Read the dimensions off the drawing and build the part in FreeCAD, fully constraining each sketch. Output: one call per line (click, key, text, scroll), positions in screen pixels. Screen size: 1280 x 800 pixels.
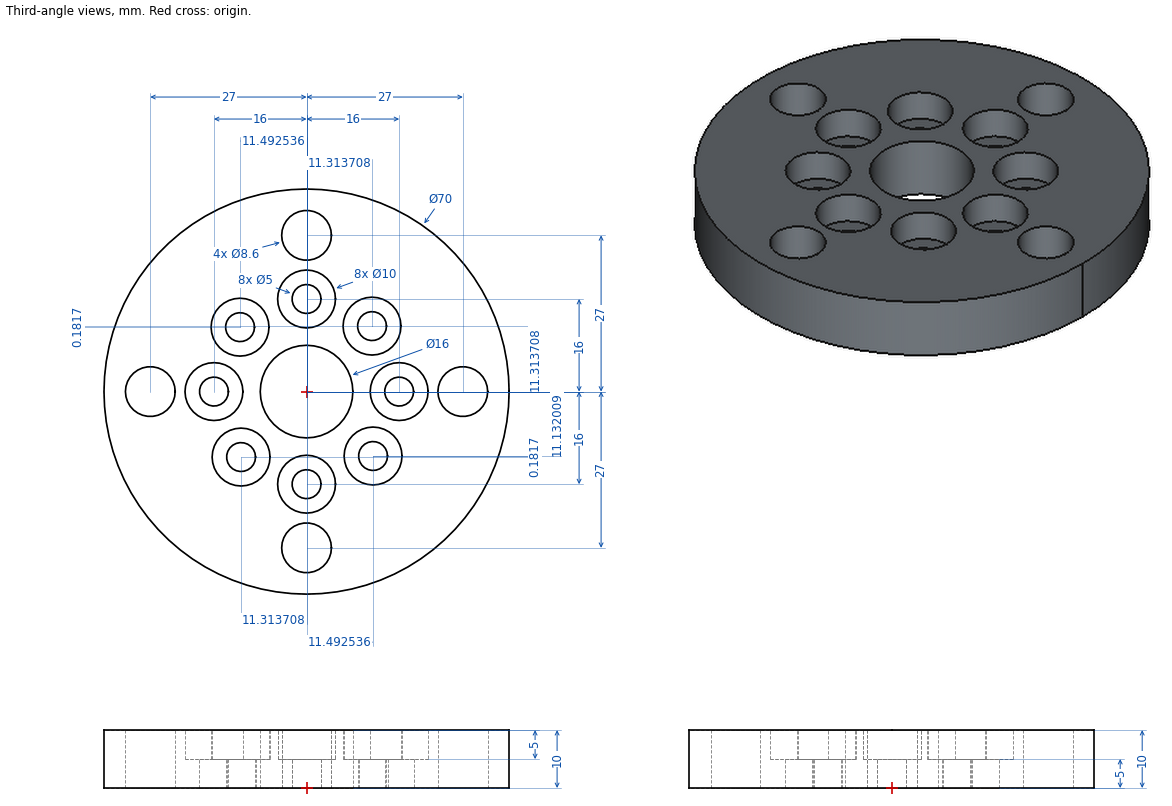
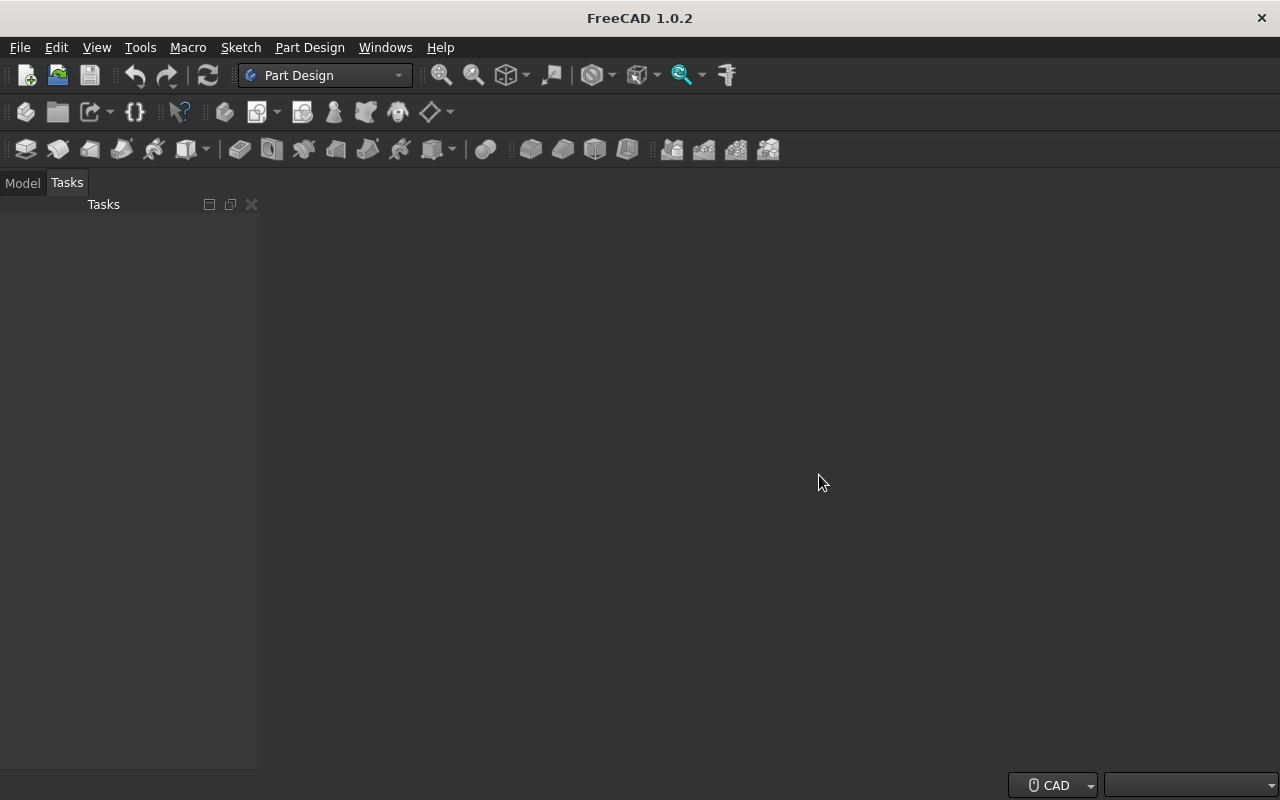
click(26, 76)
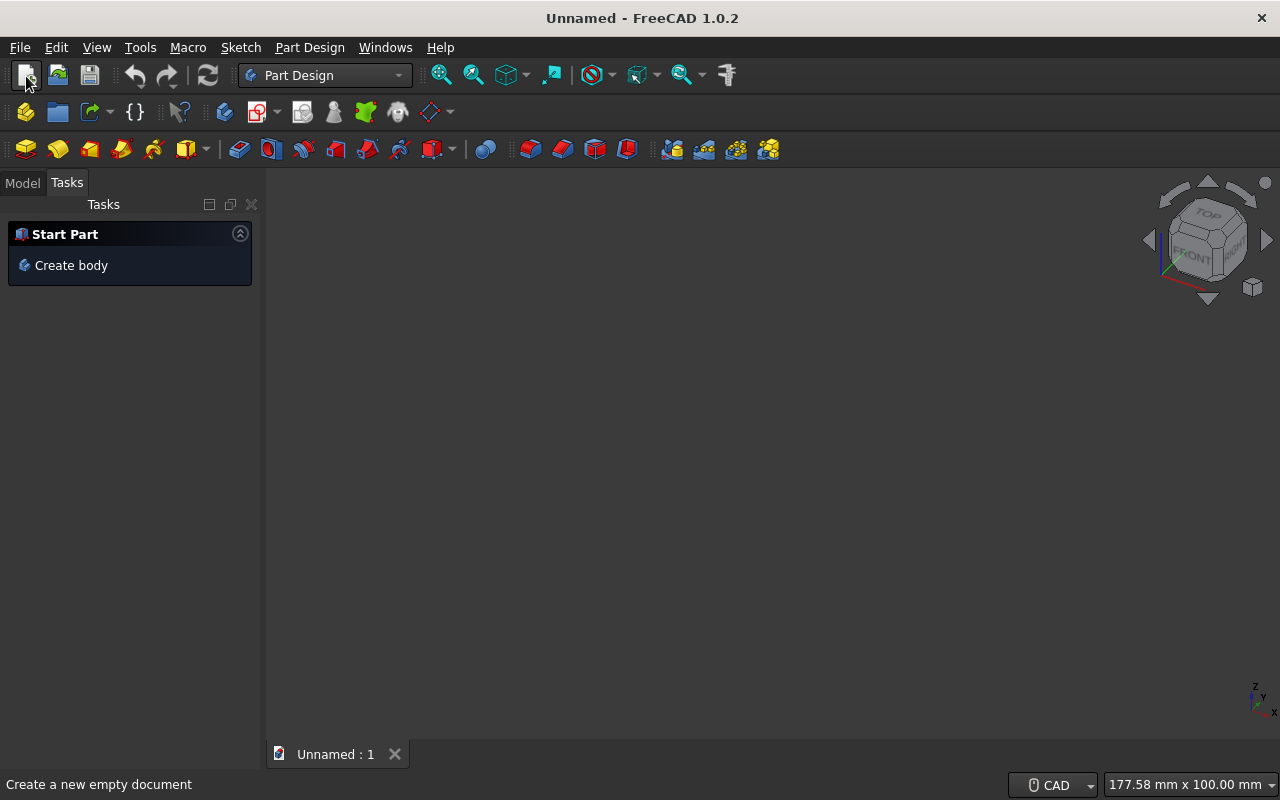
click(258, 112)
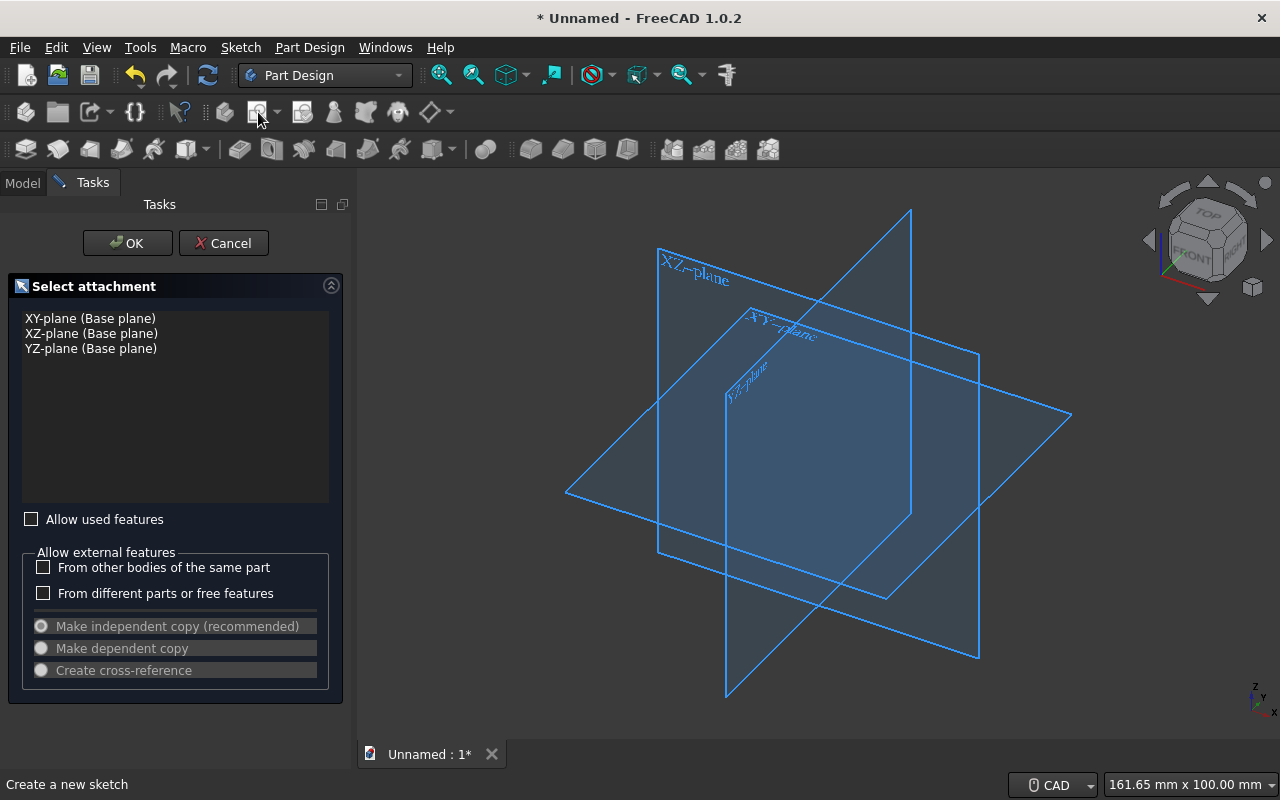
click(82, 318)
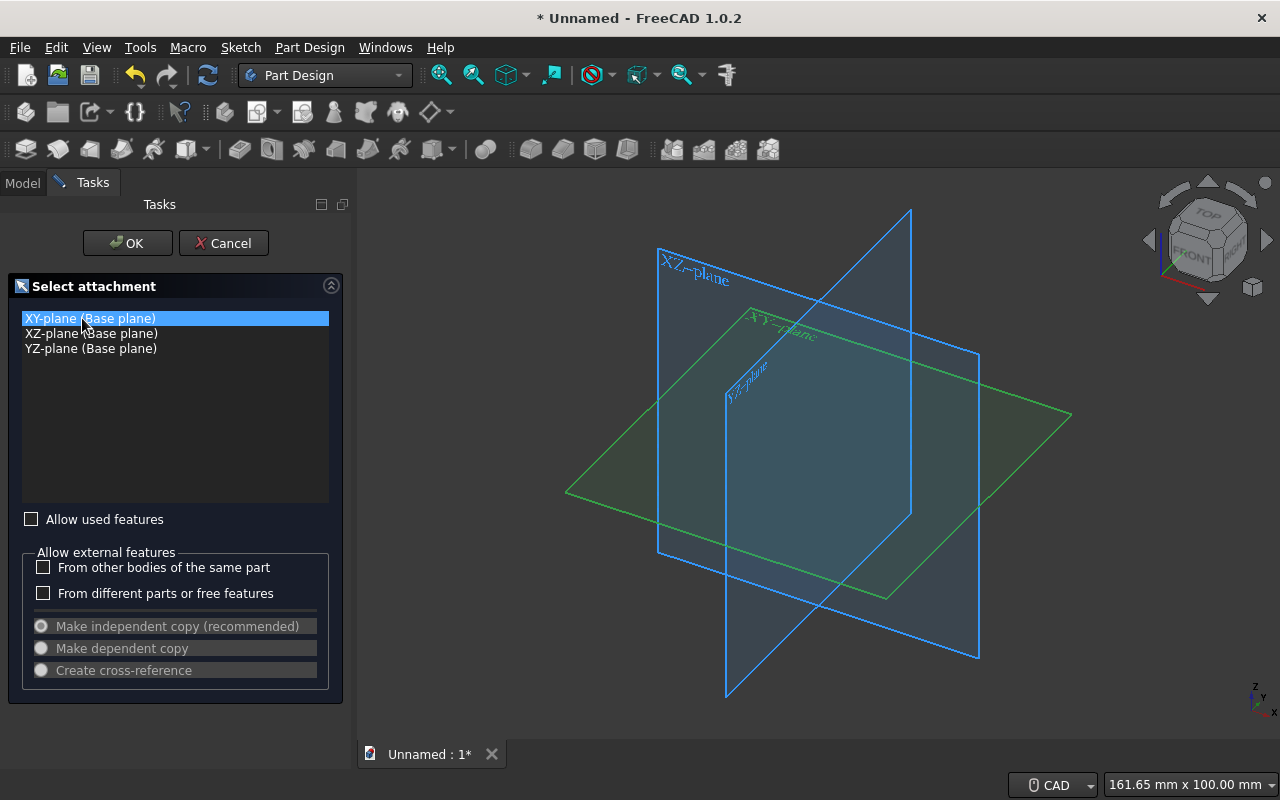
click(128, 243)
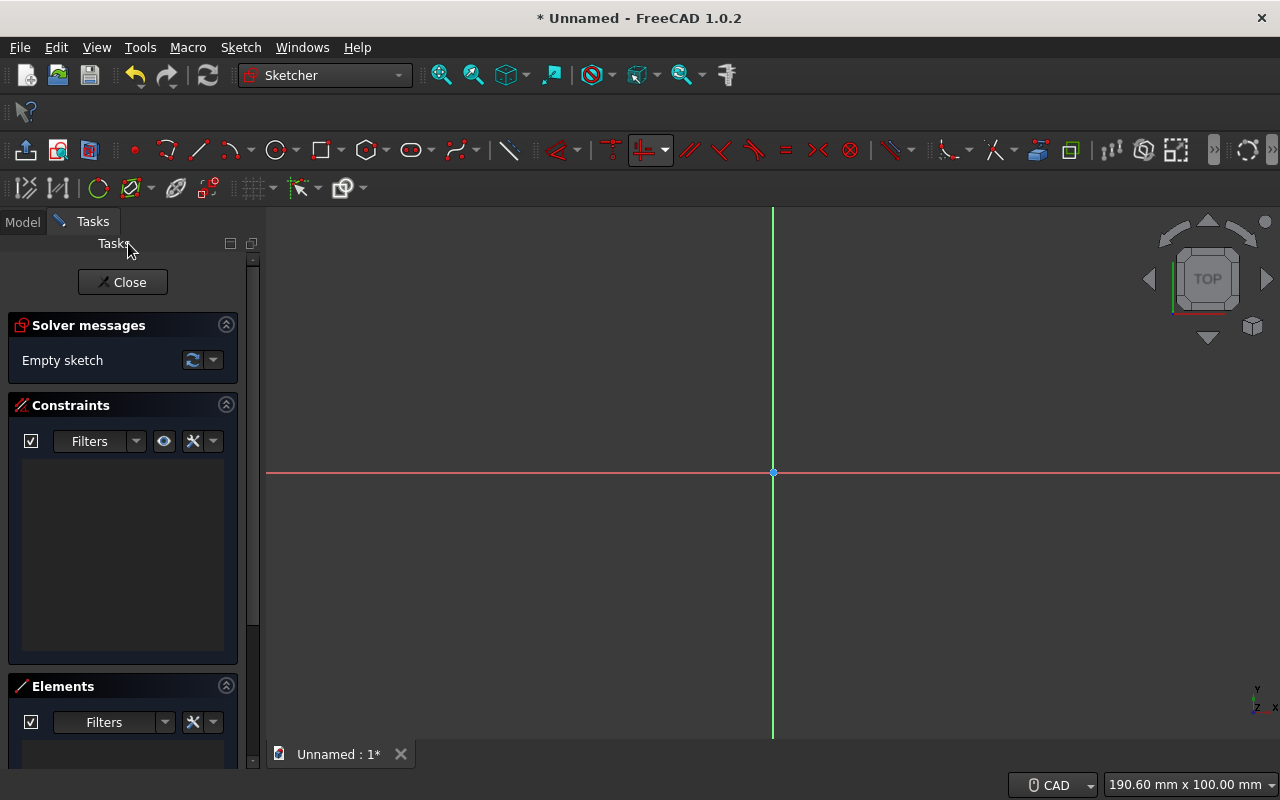
click(276, 150)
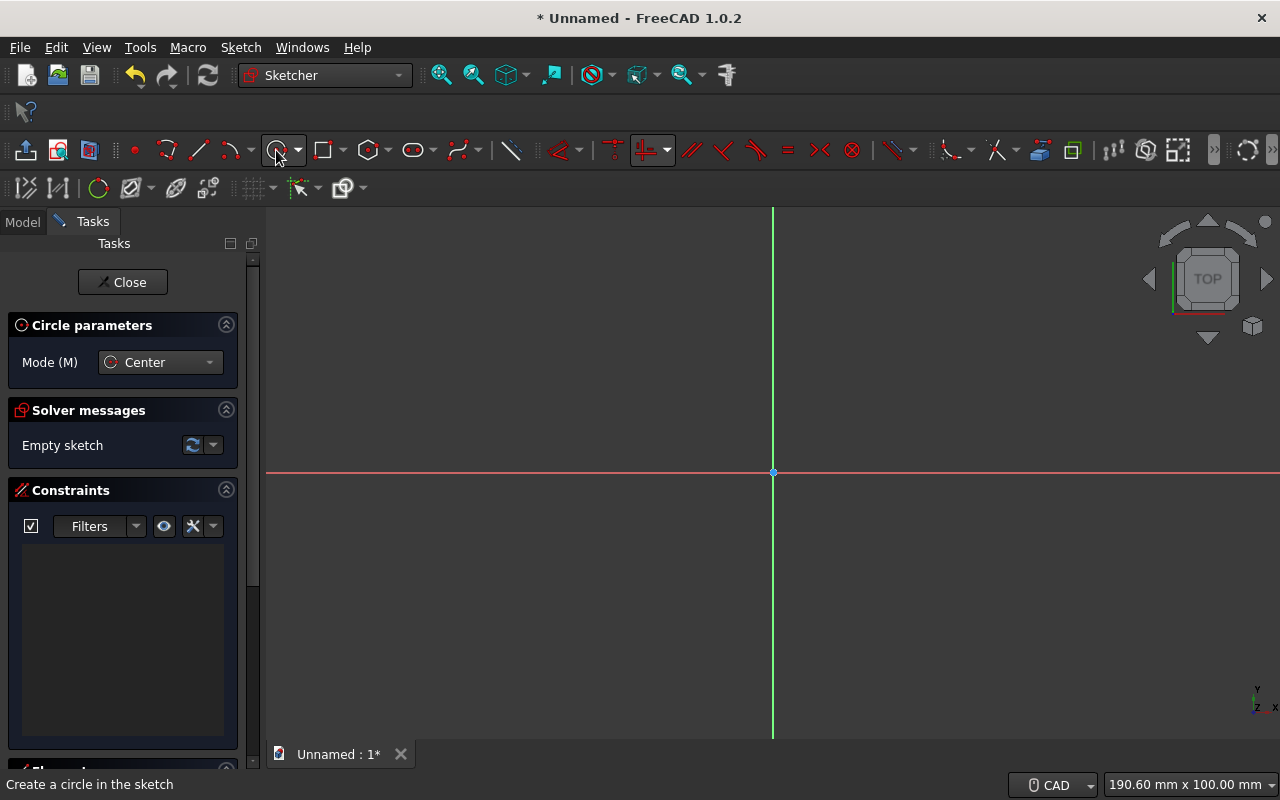
click(773, 473)
move(905, 341)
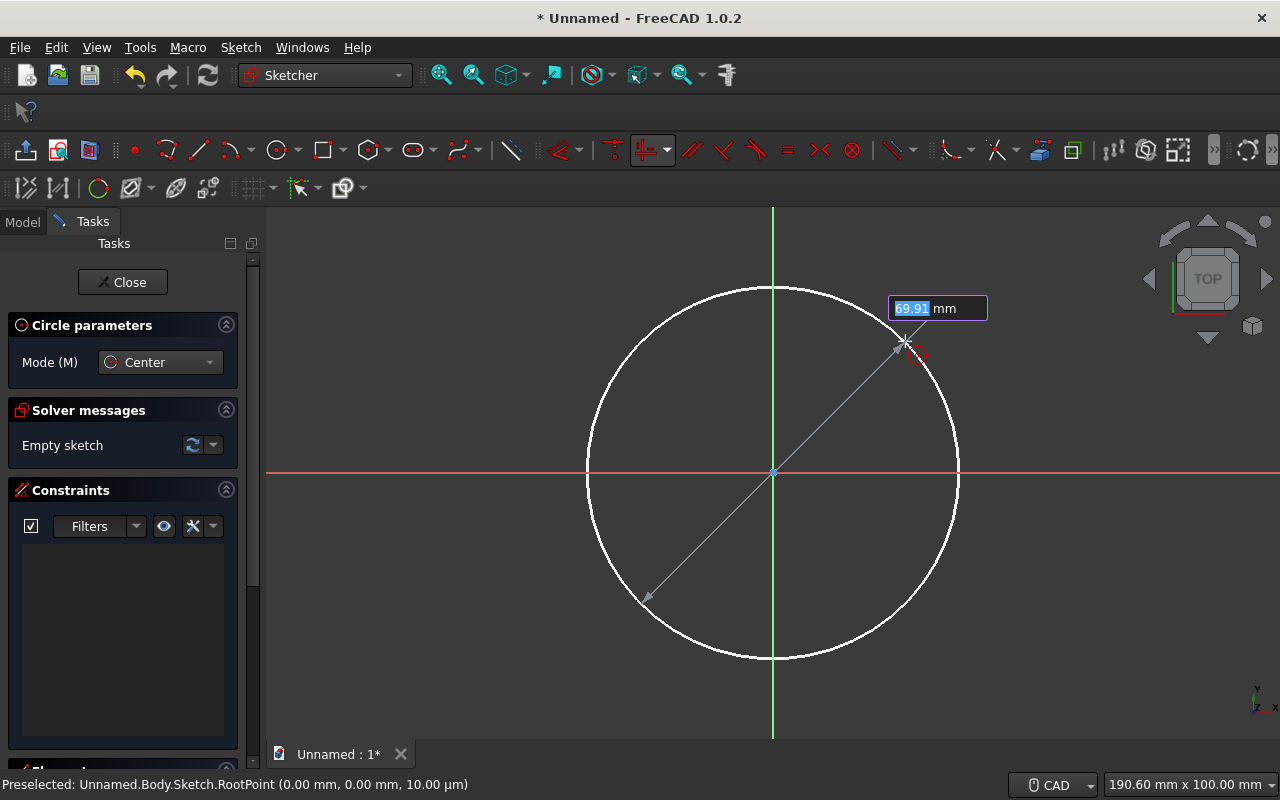
text(70)
key(Return)
key(Escape)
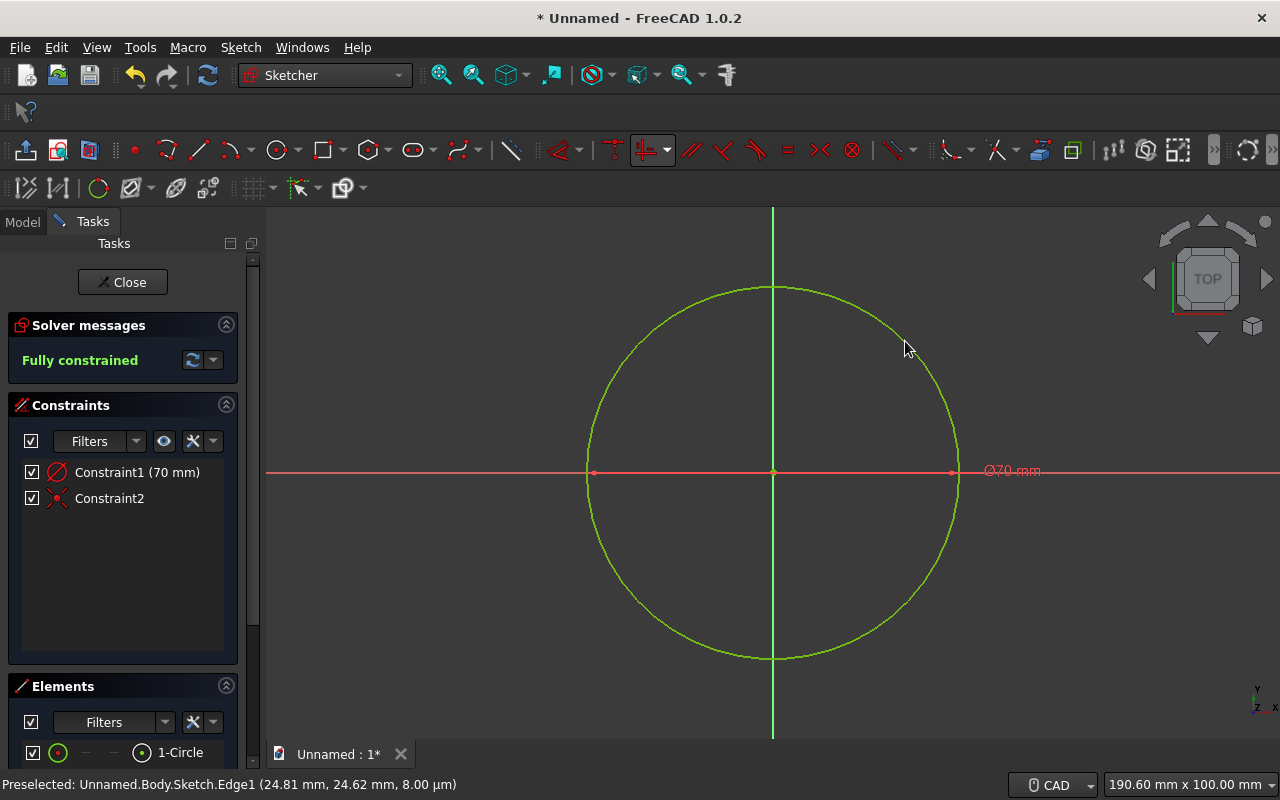
click(123, 282)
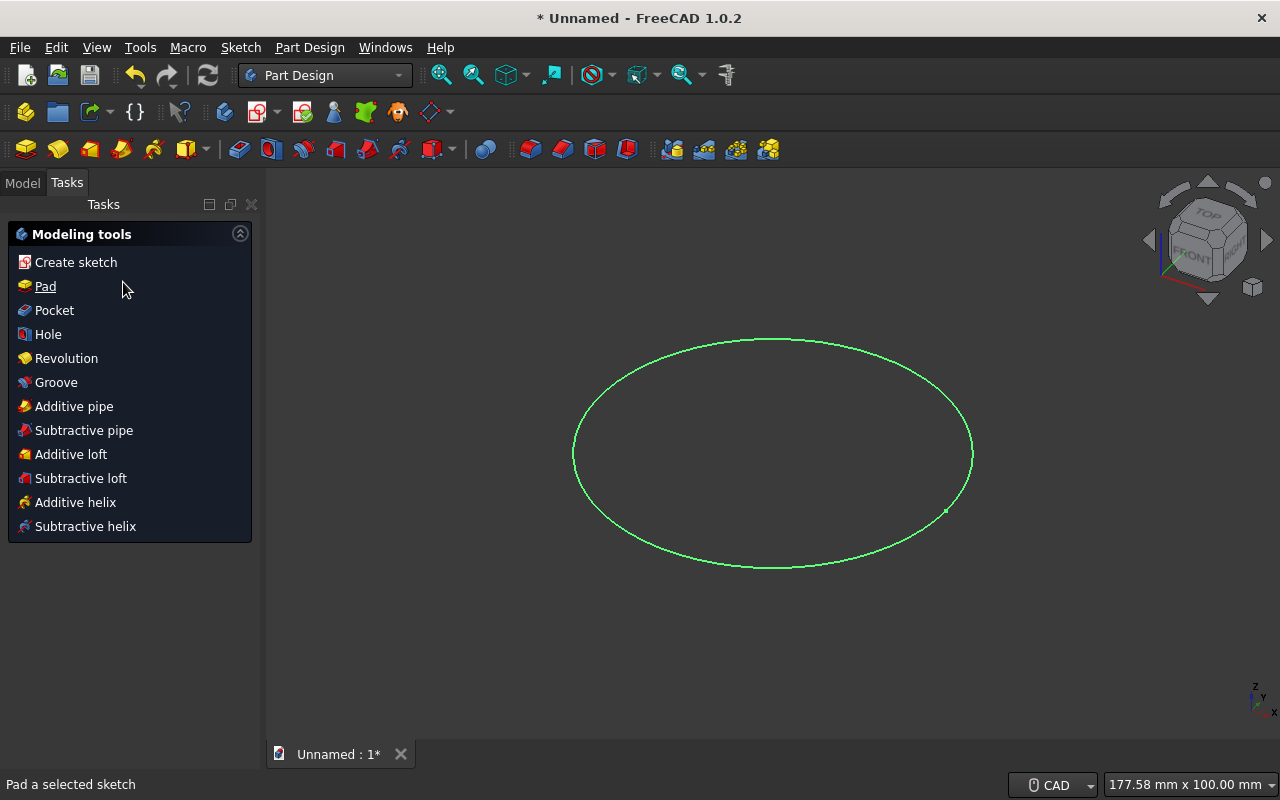
click(26, 150)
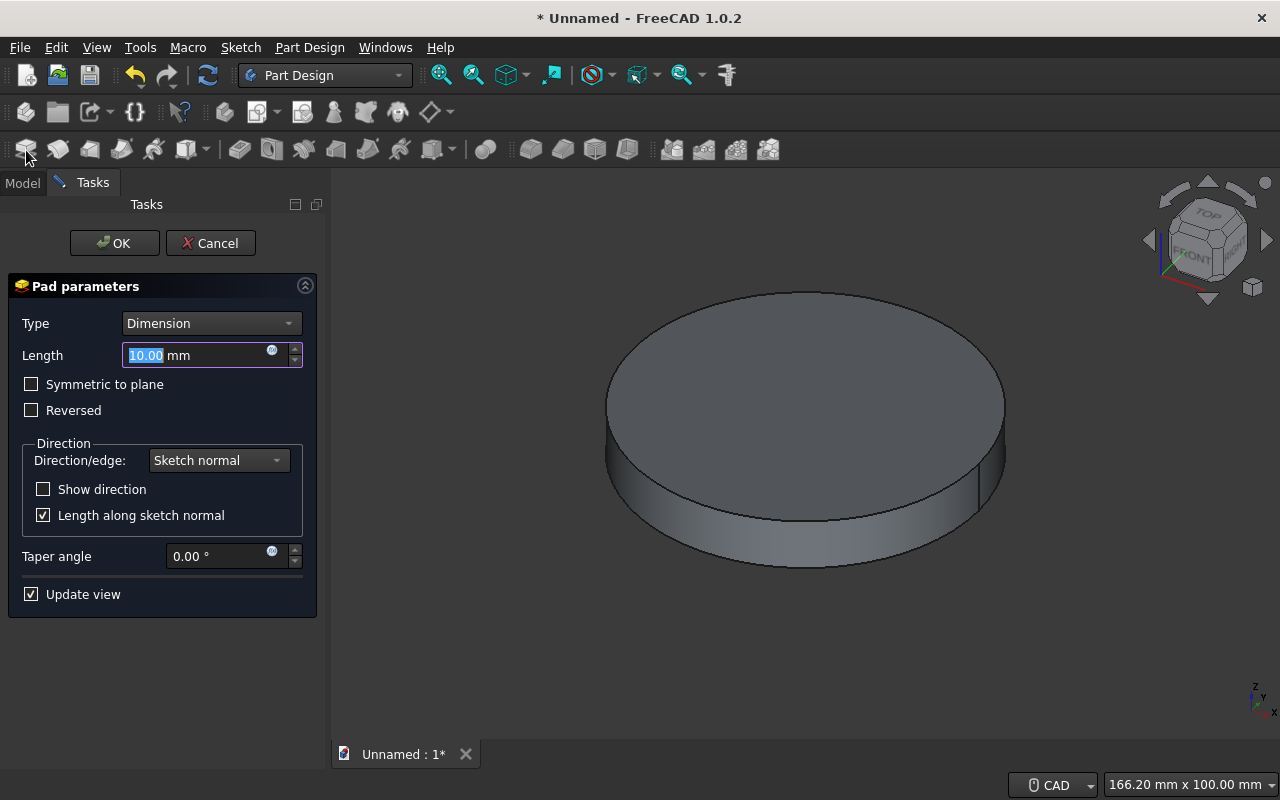
text(10)
key(Tab)